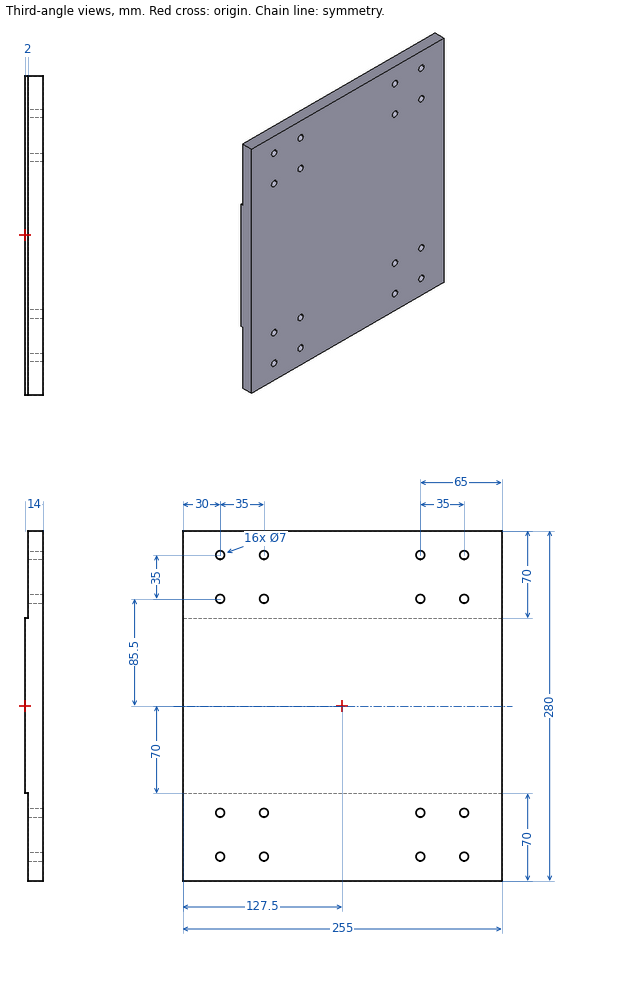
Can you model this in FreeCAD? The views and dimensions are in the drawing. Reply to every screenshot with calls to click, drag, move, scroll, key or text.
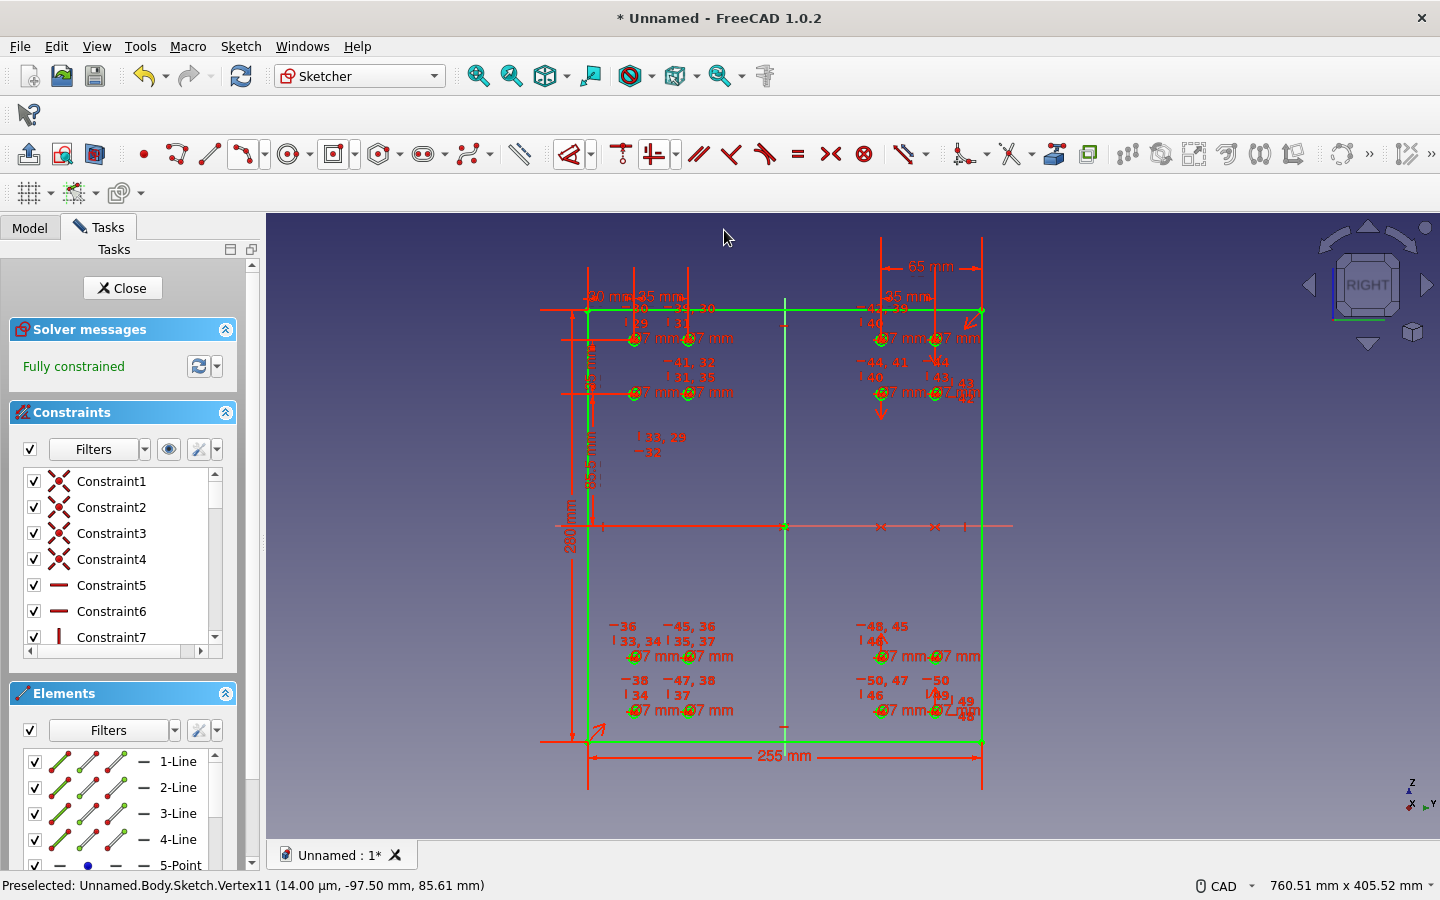
click(123, 288)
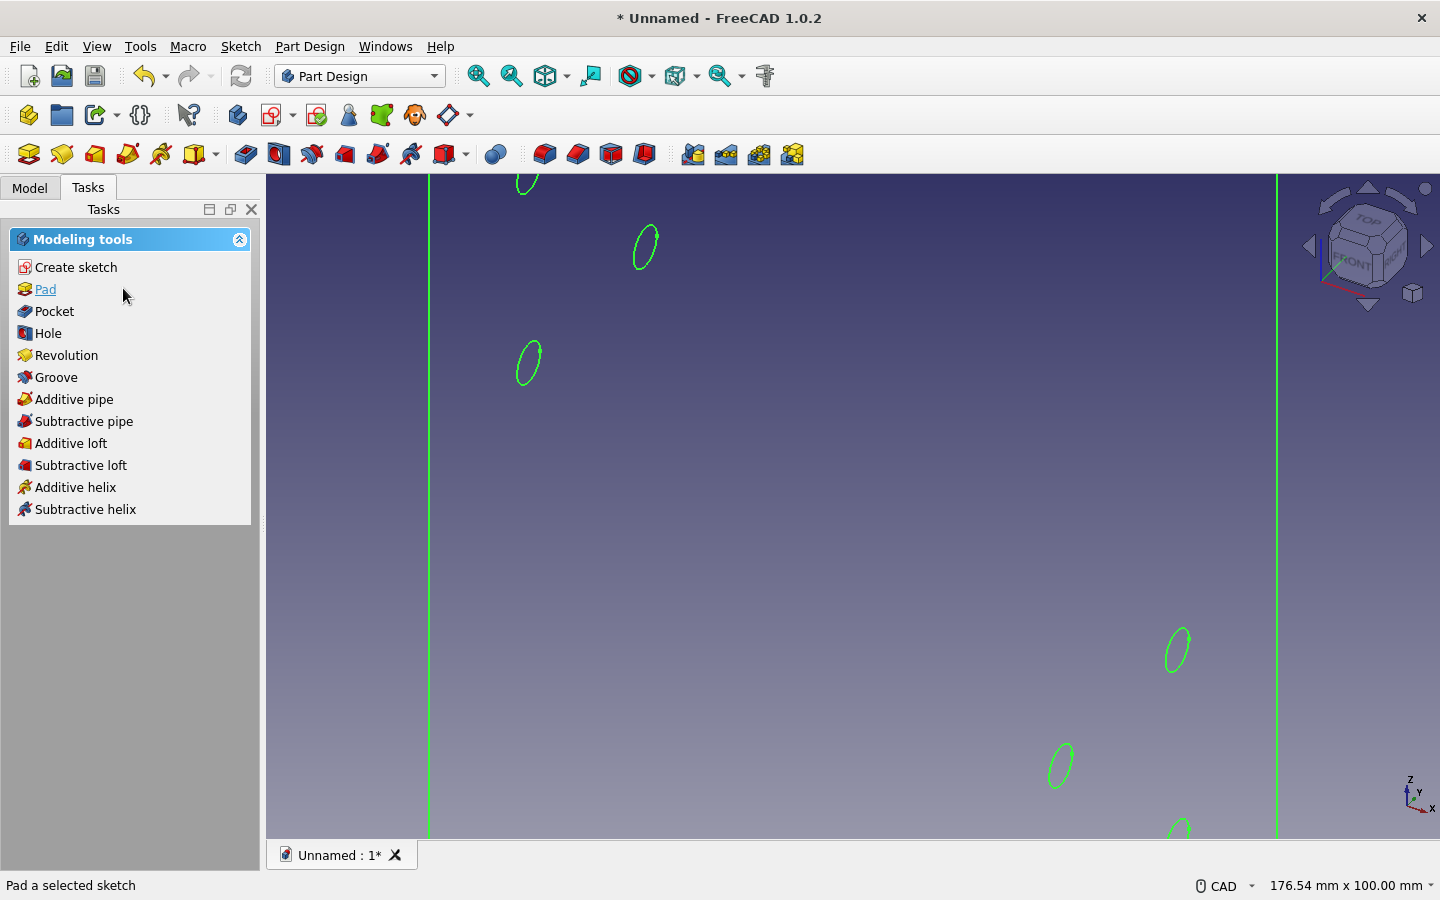
click(29, 154)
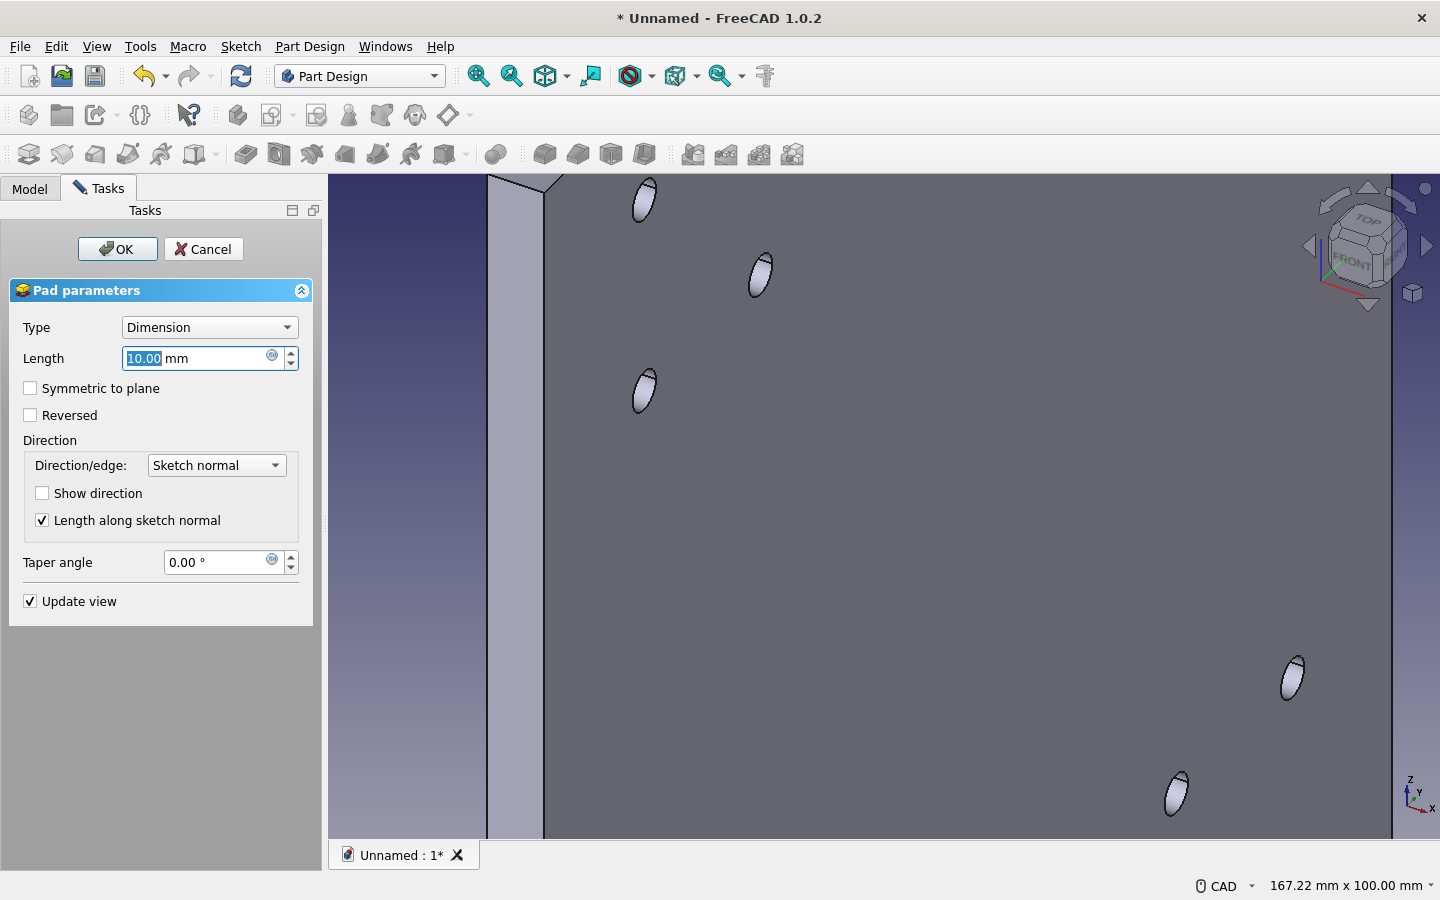
text(14)
key(Tab)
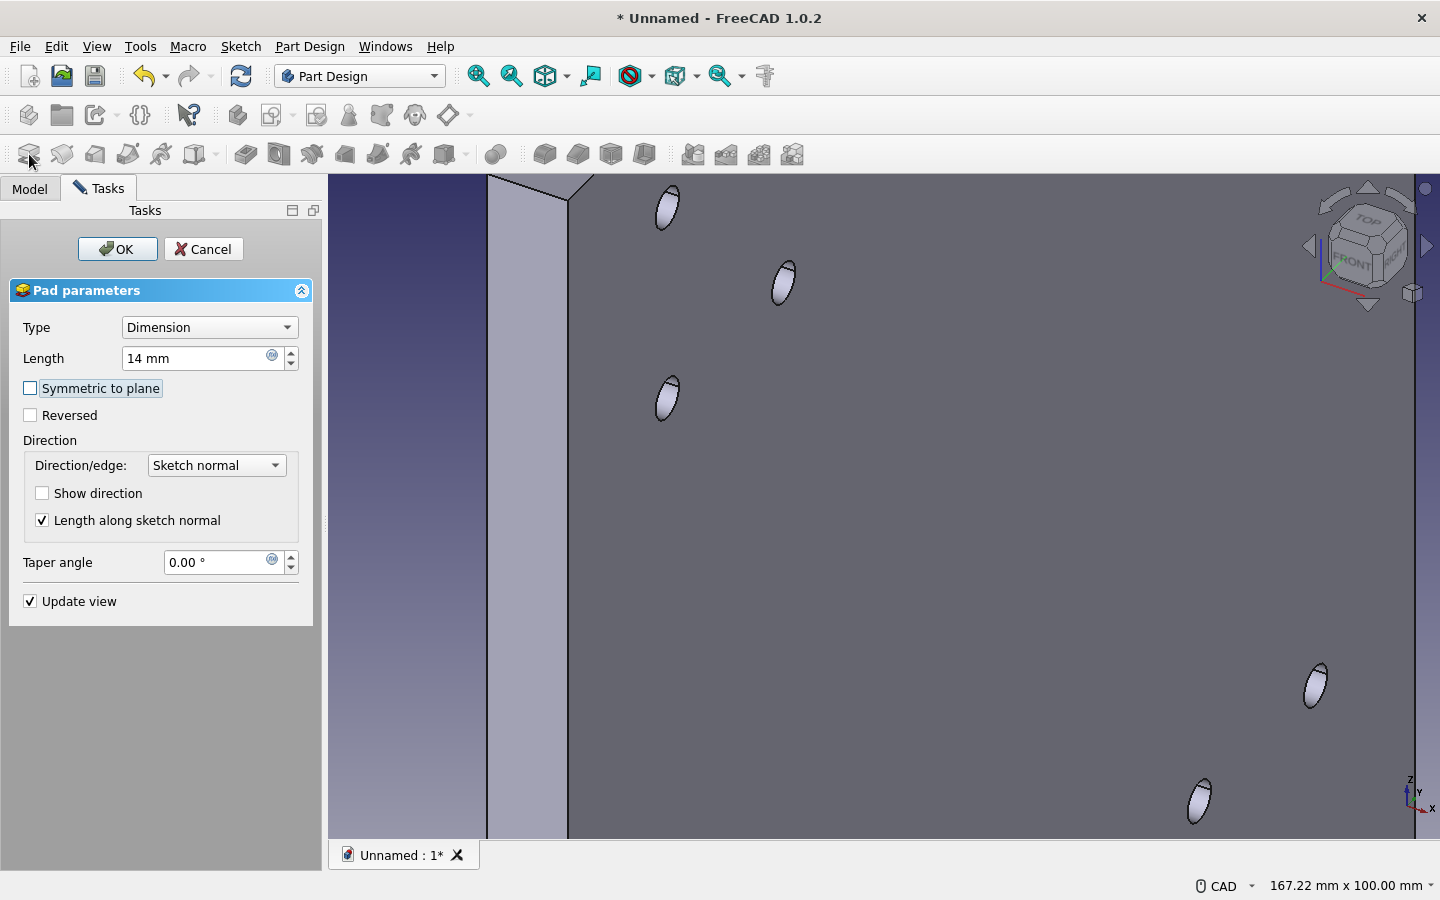
click(118, 249)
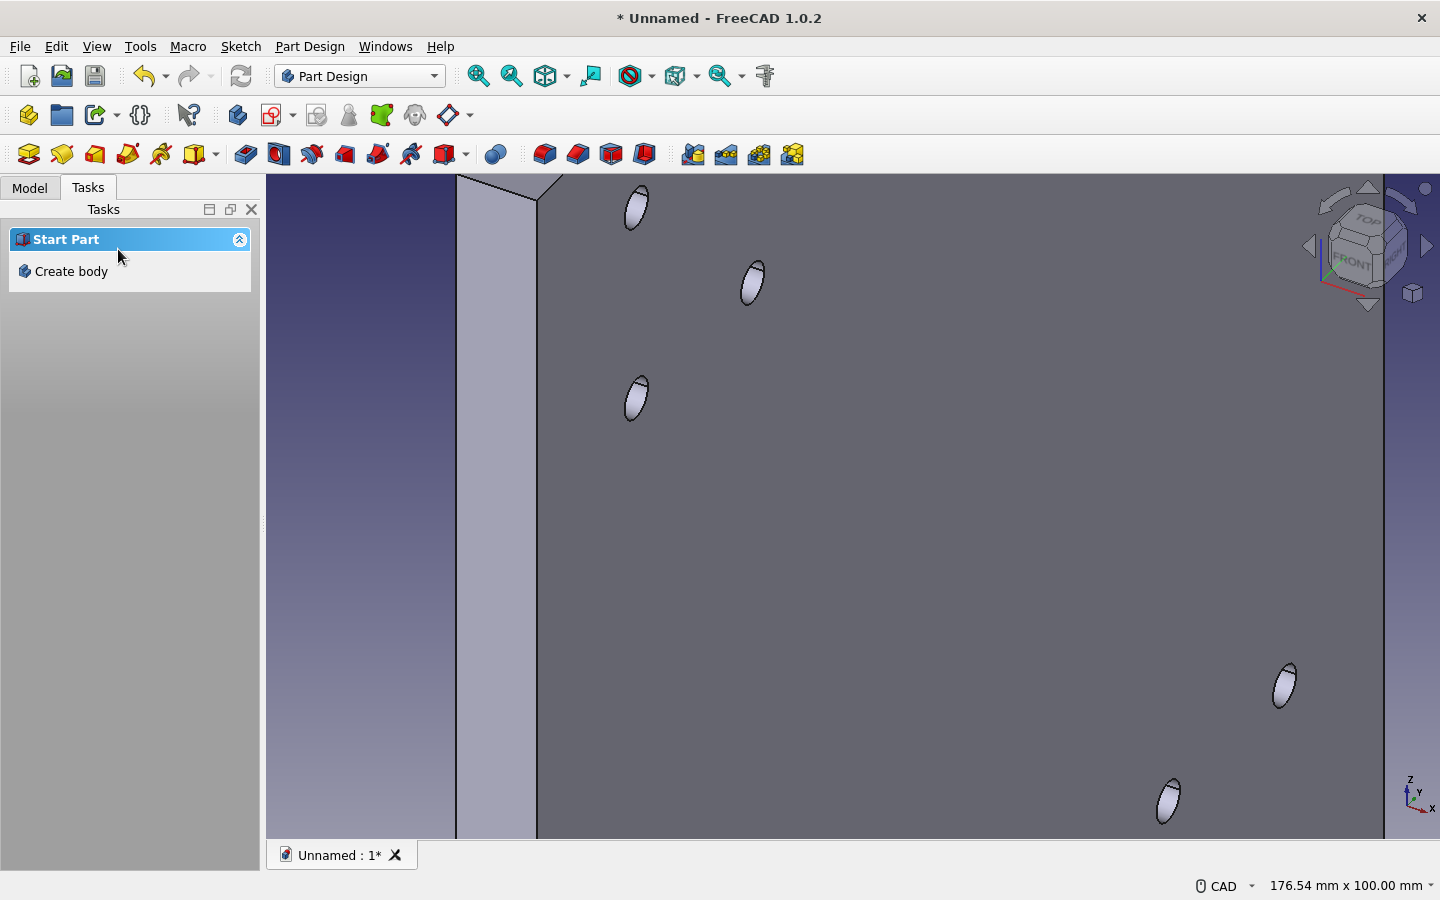
click(479, 76)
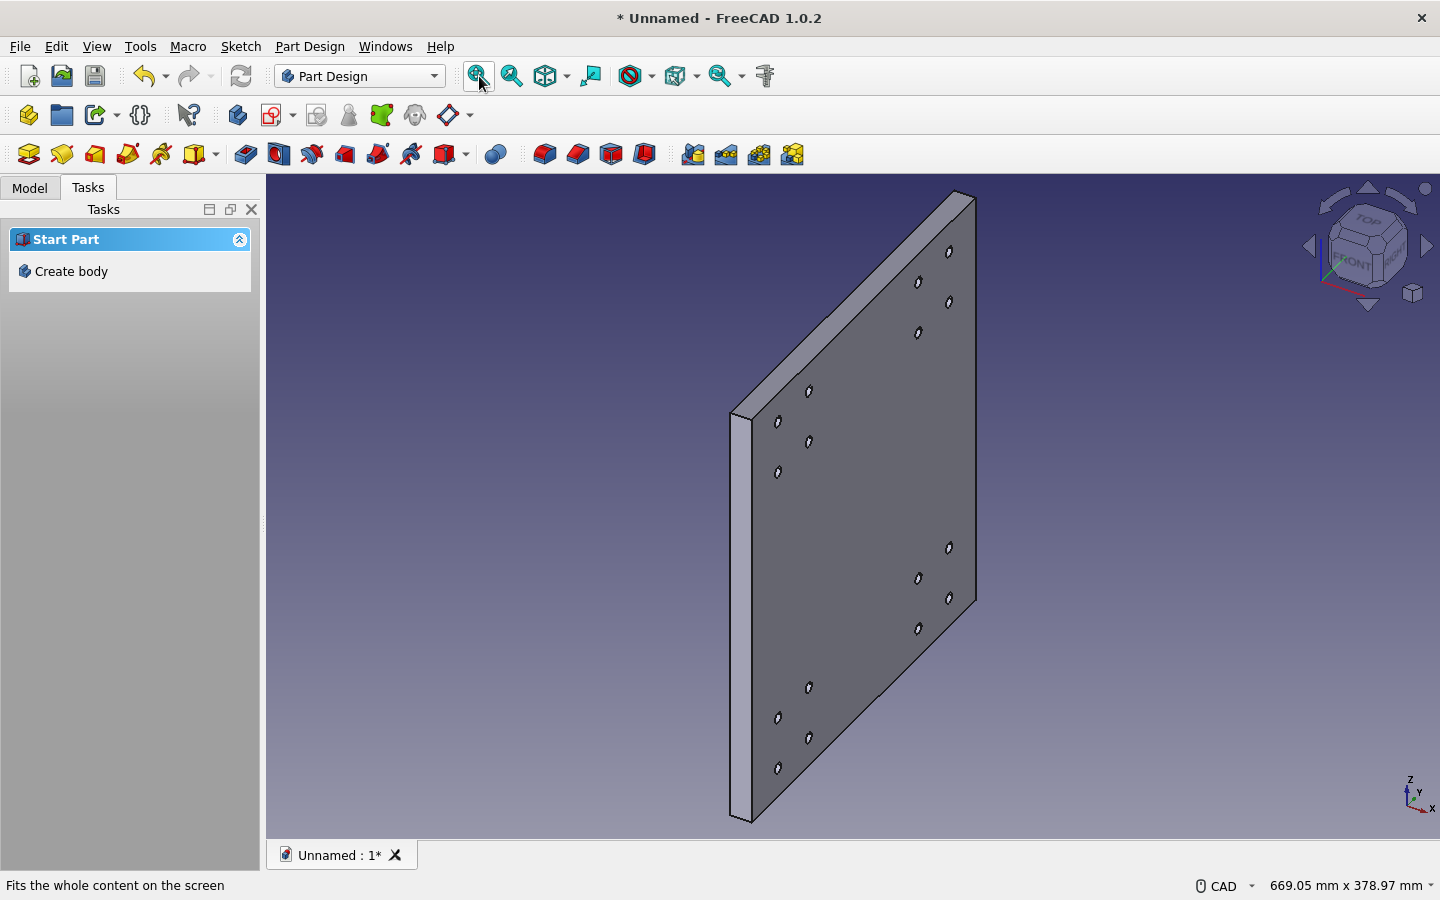
click(270, 116)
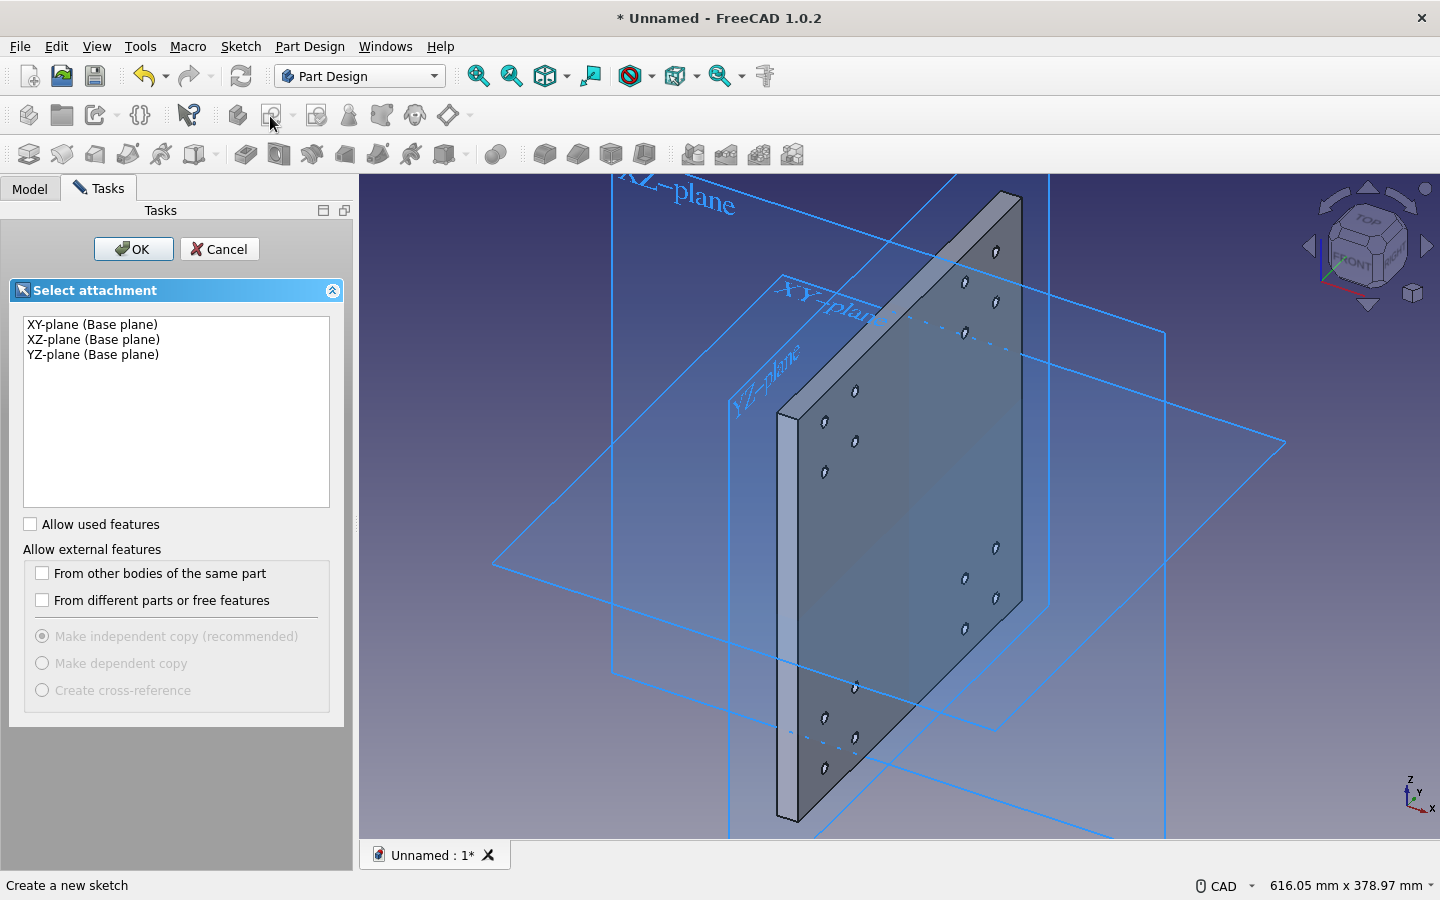
click(84, 354)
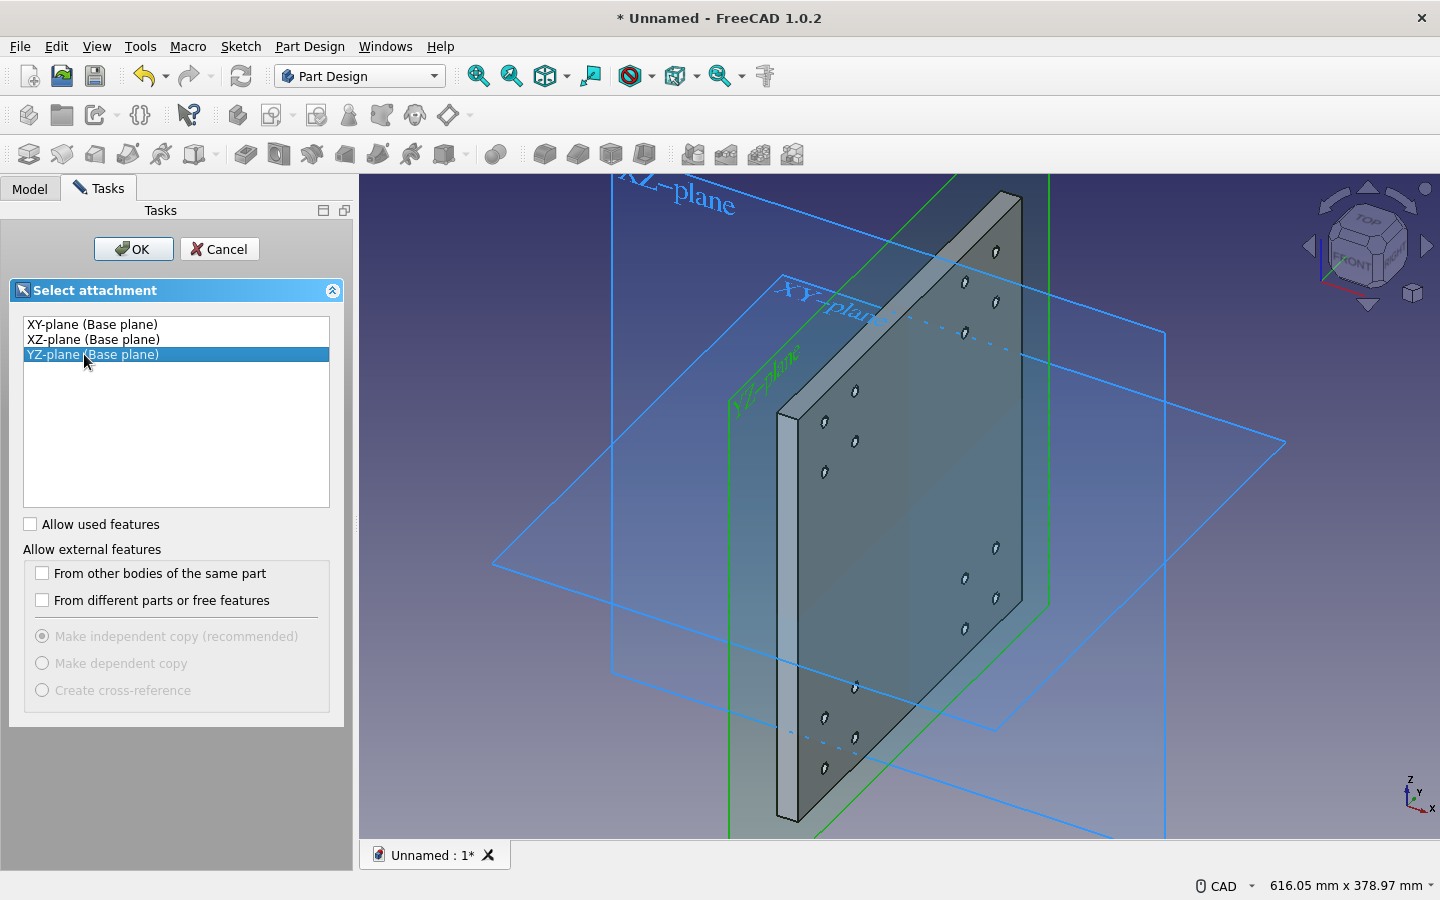
click(134, 249)